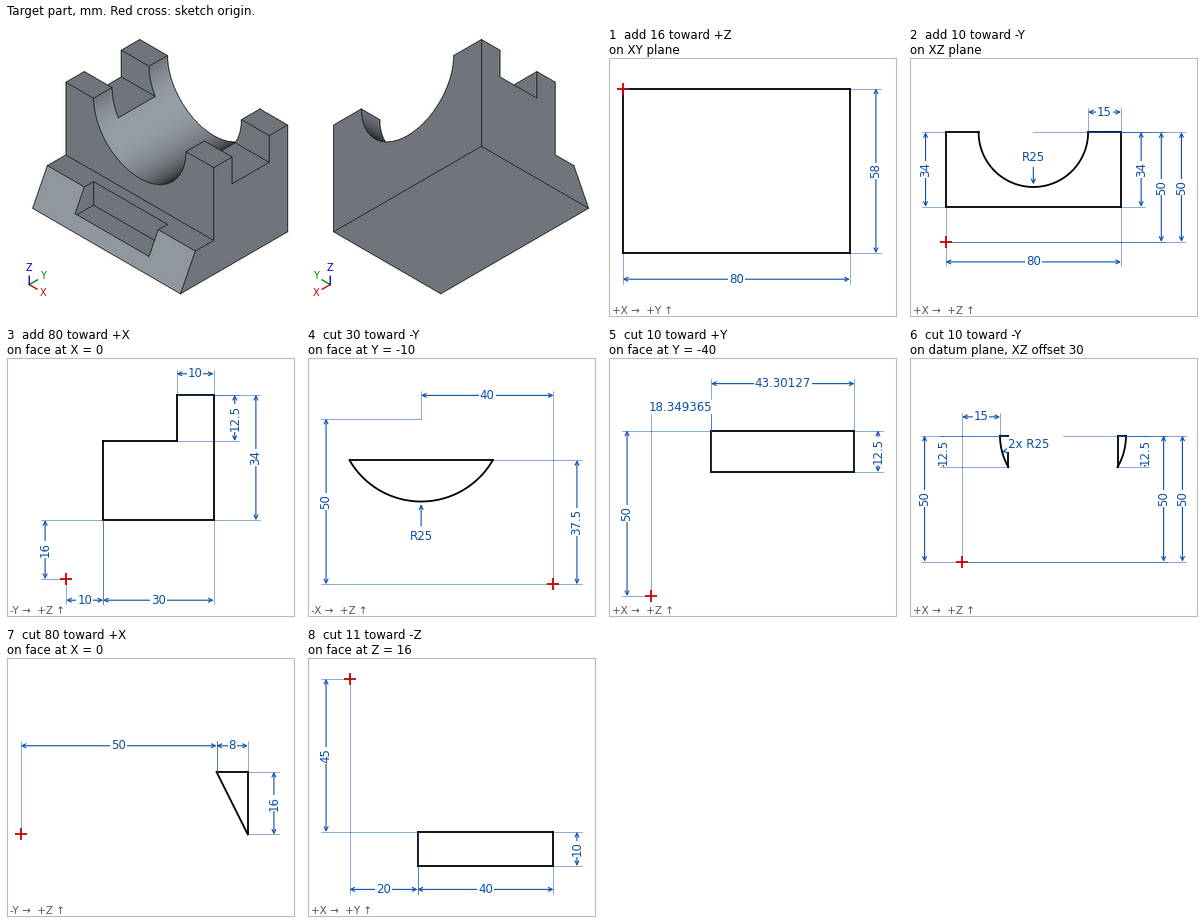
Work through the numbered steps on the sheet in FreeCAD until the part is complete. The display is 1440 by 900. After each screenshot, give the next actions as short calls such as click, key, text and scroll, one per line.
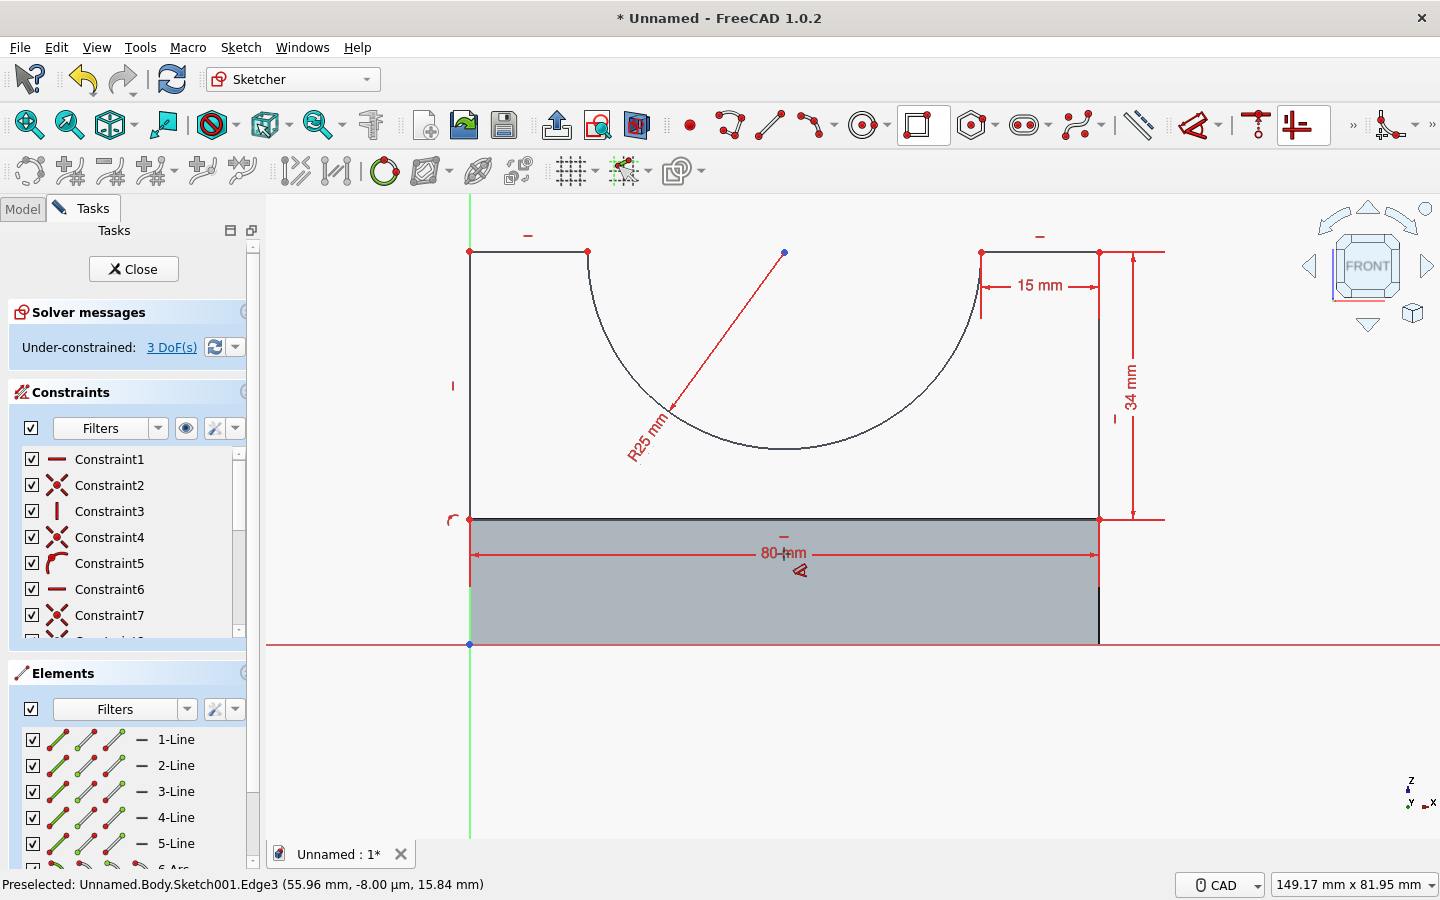
click(470, 440)
click(436, 386)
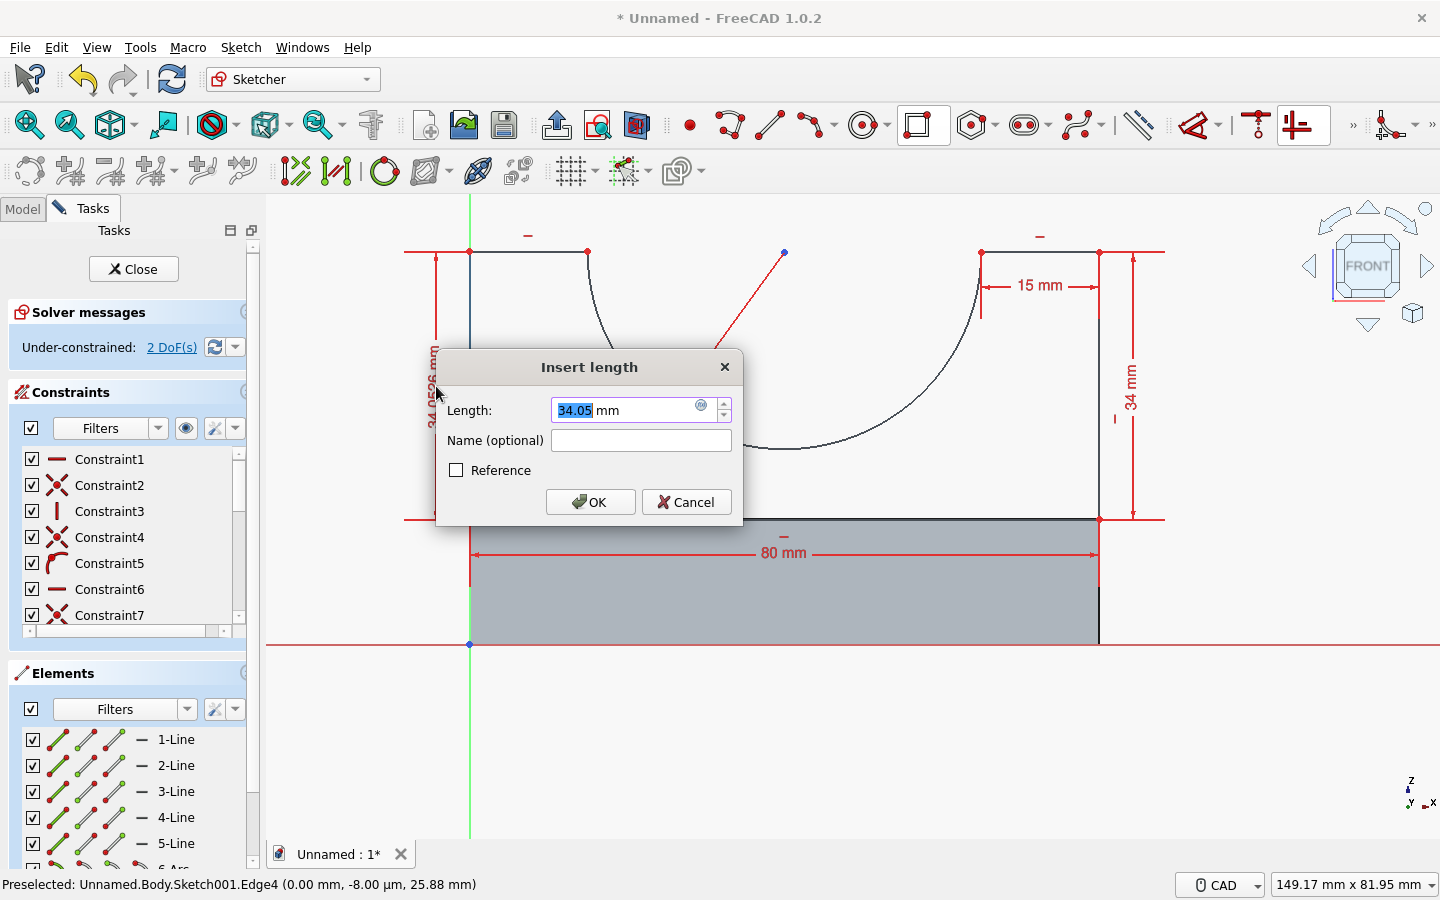
text(34)
key(Return)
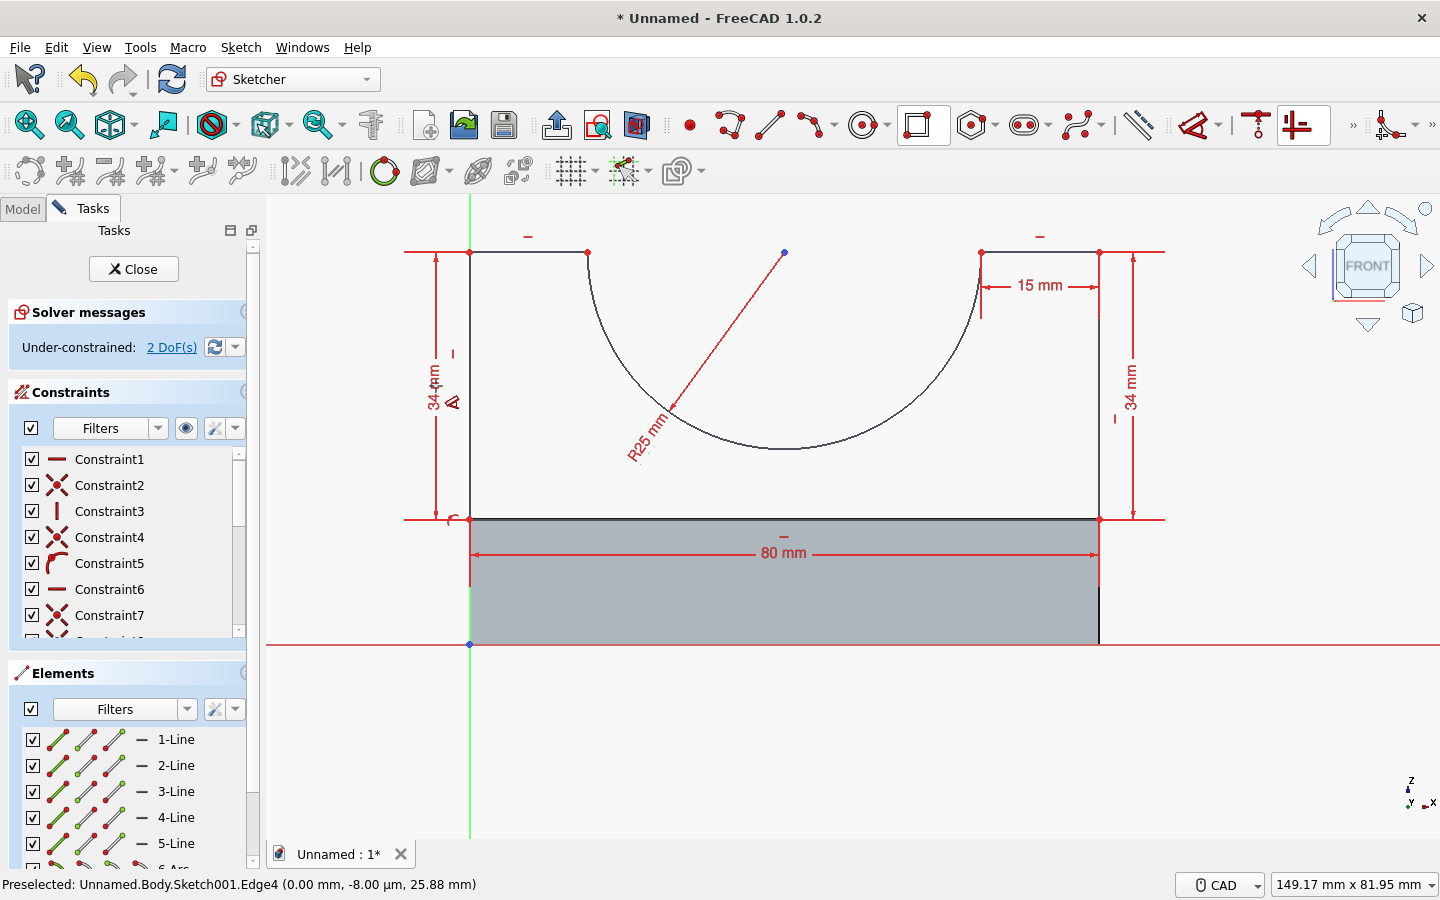
click(981, 252)
click(436, 449)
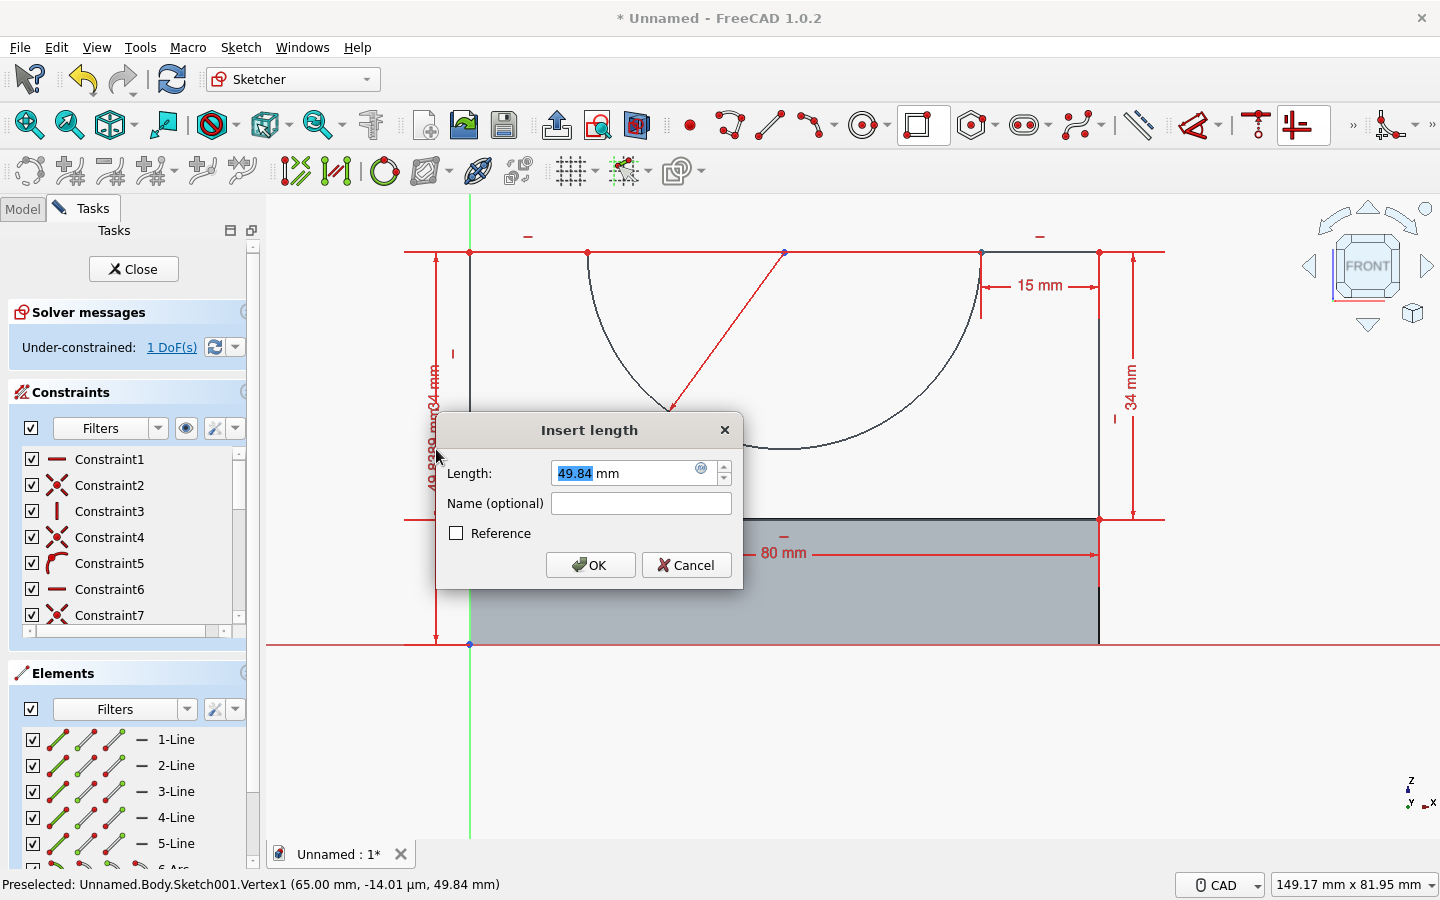
text(50)
key(Return)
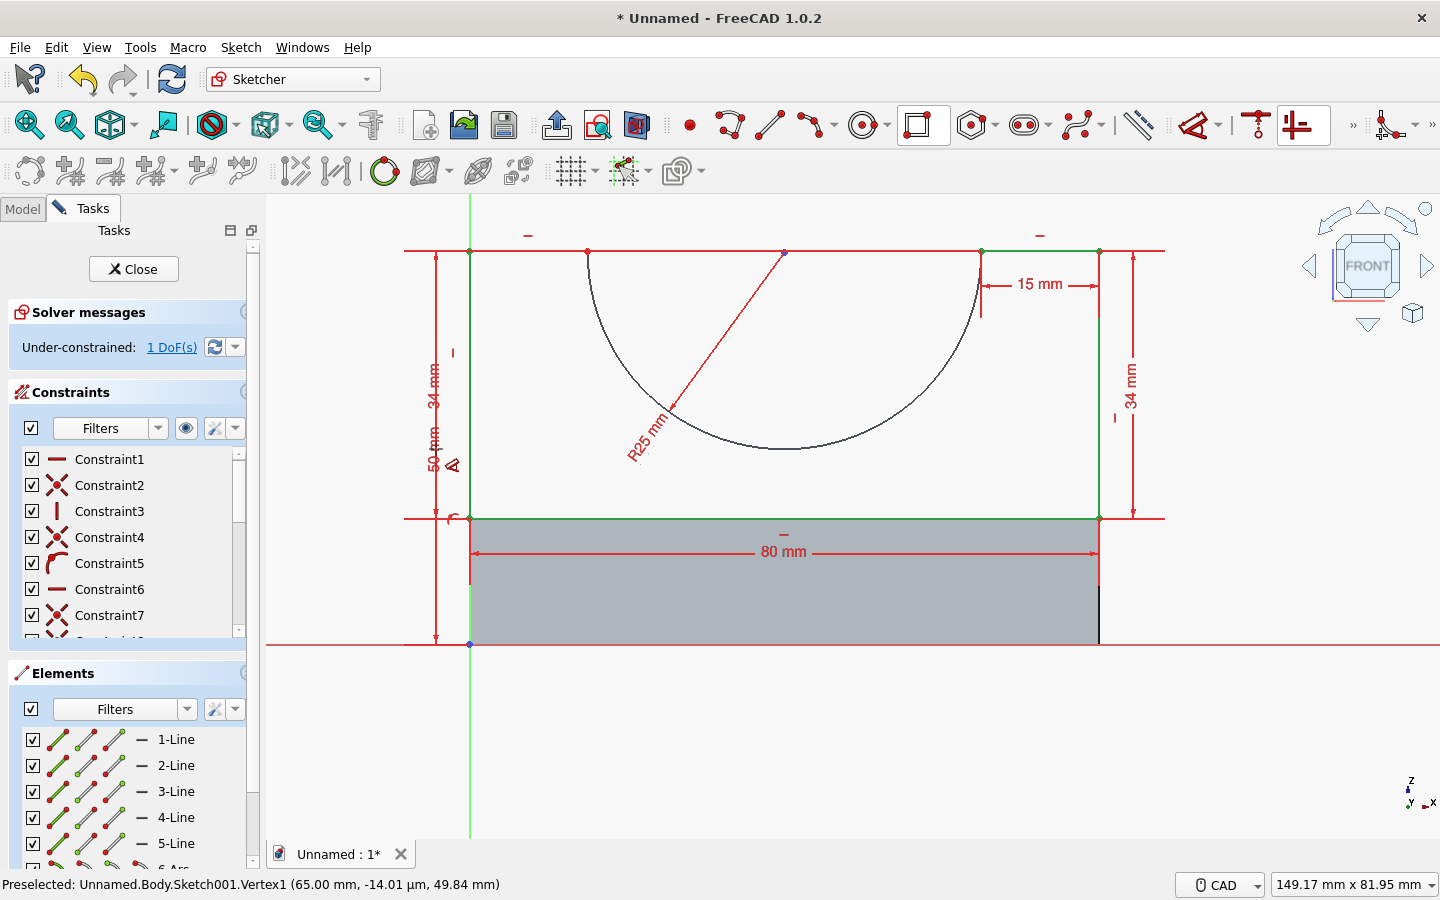
click(784, 253)
click(436, 358)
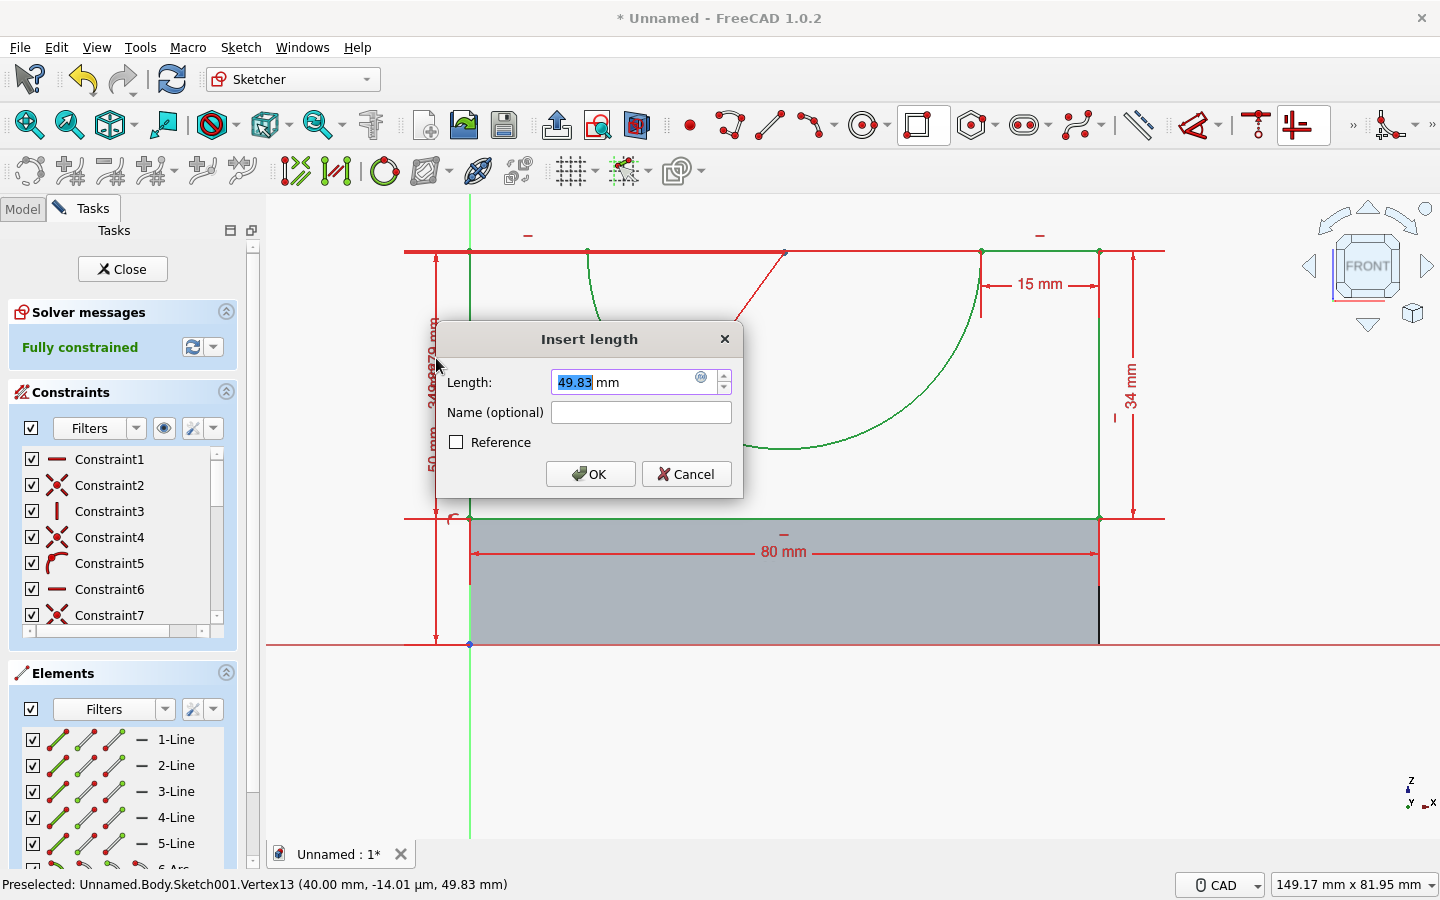
text(50)
key(Return)
key(Escape)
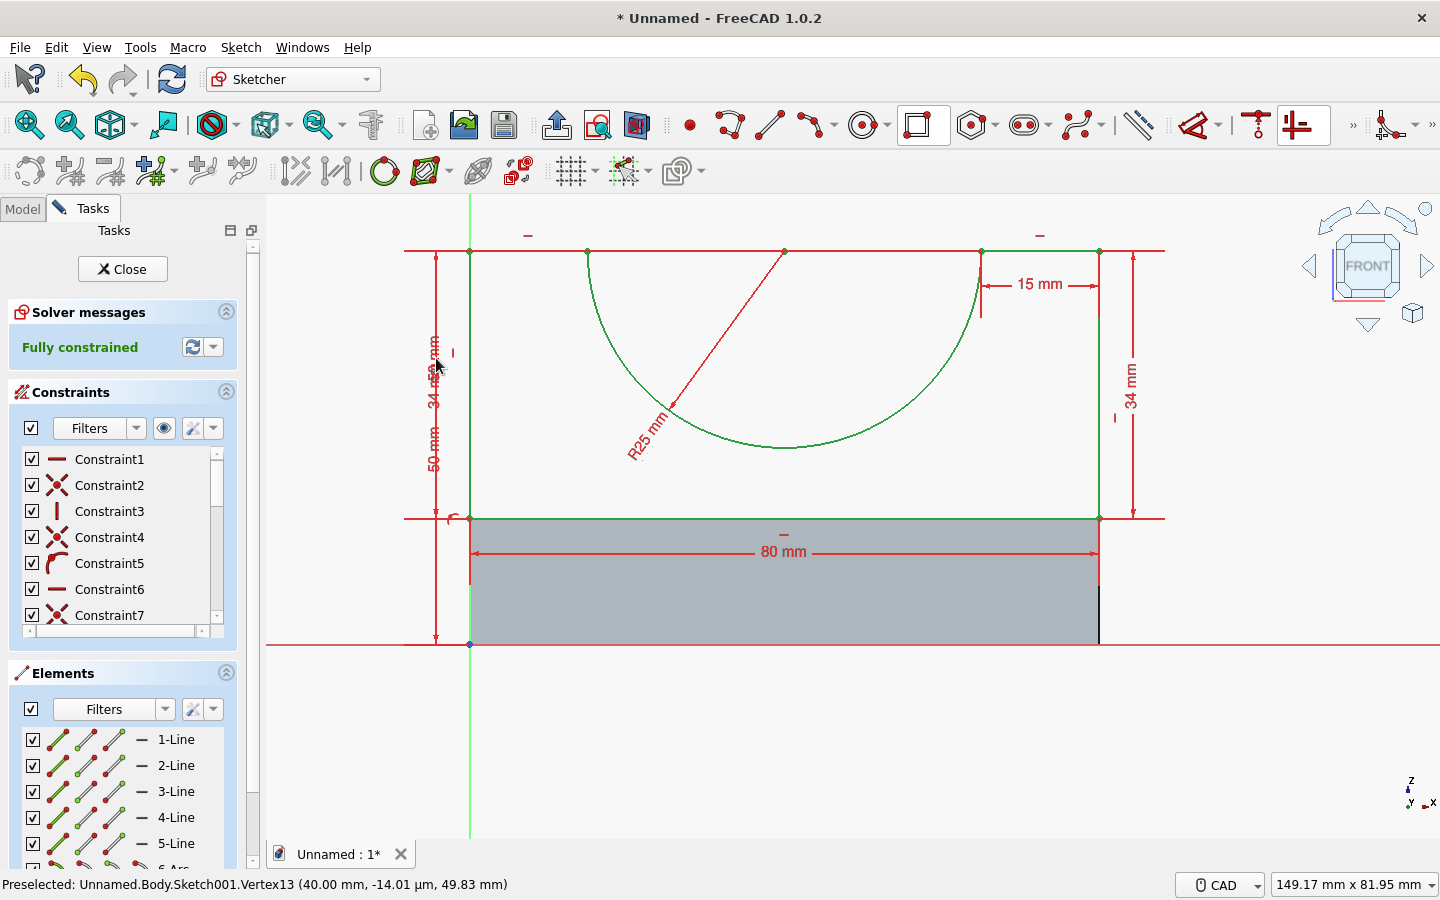
click(123, 269)